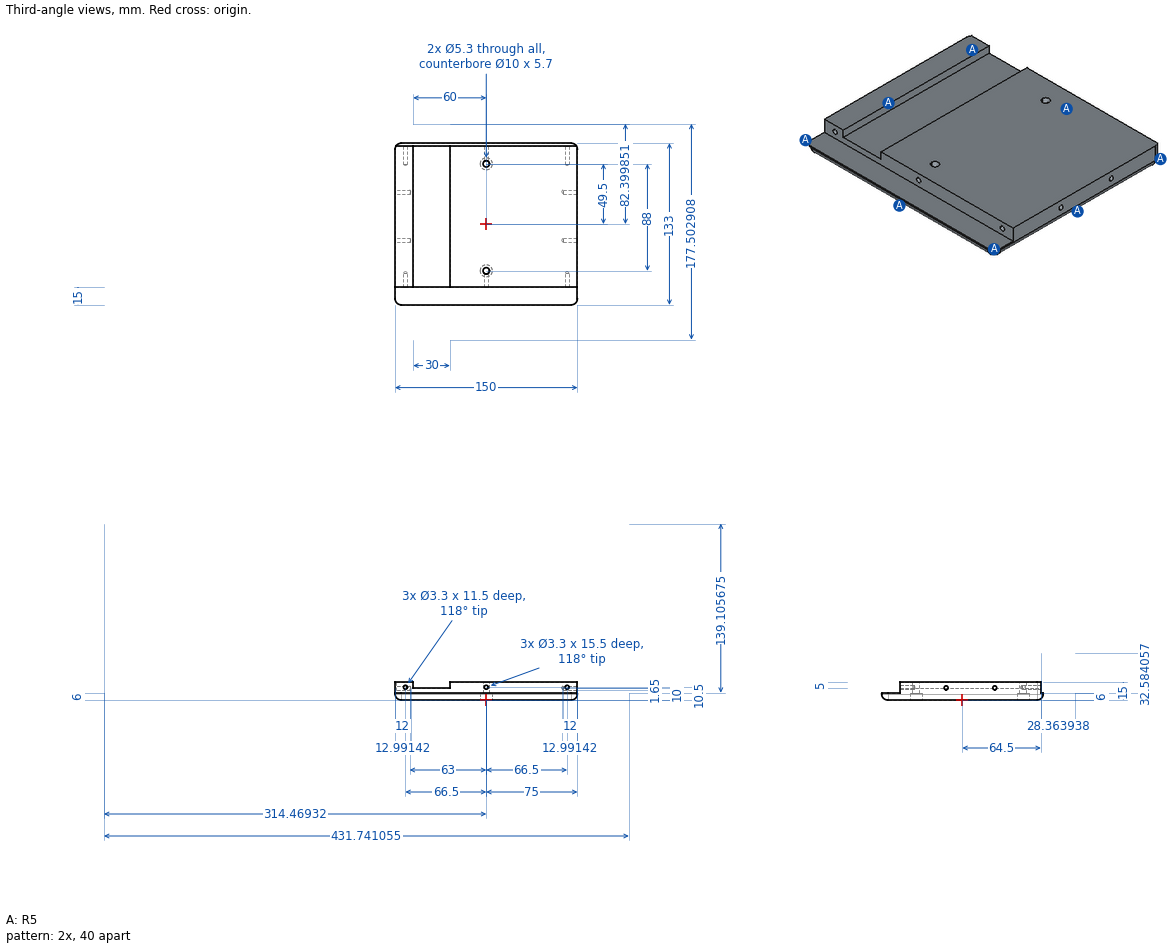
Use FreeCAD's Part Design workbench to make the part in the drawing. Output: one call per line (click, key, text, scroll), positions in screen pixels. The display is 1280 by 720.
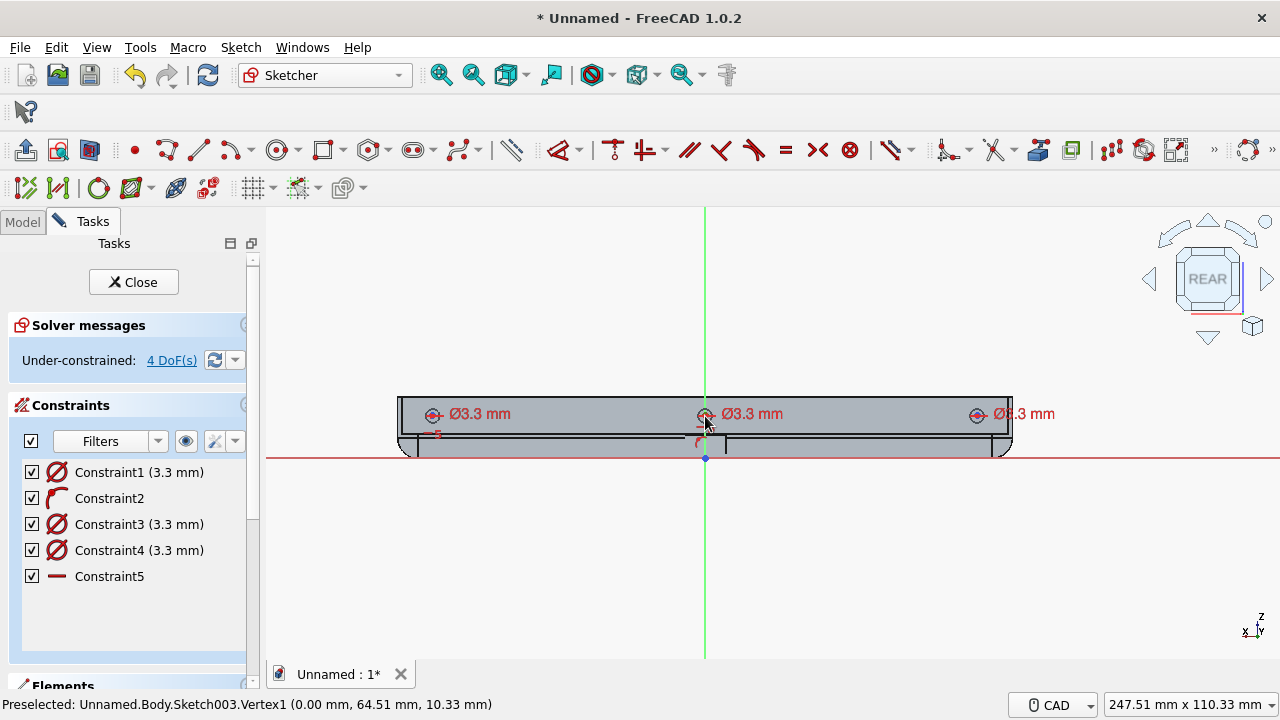
click(977, 416)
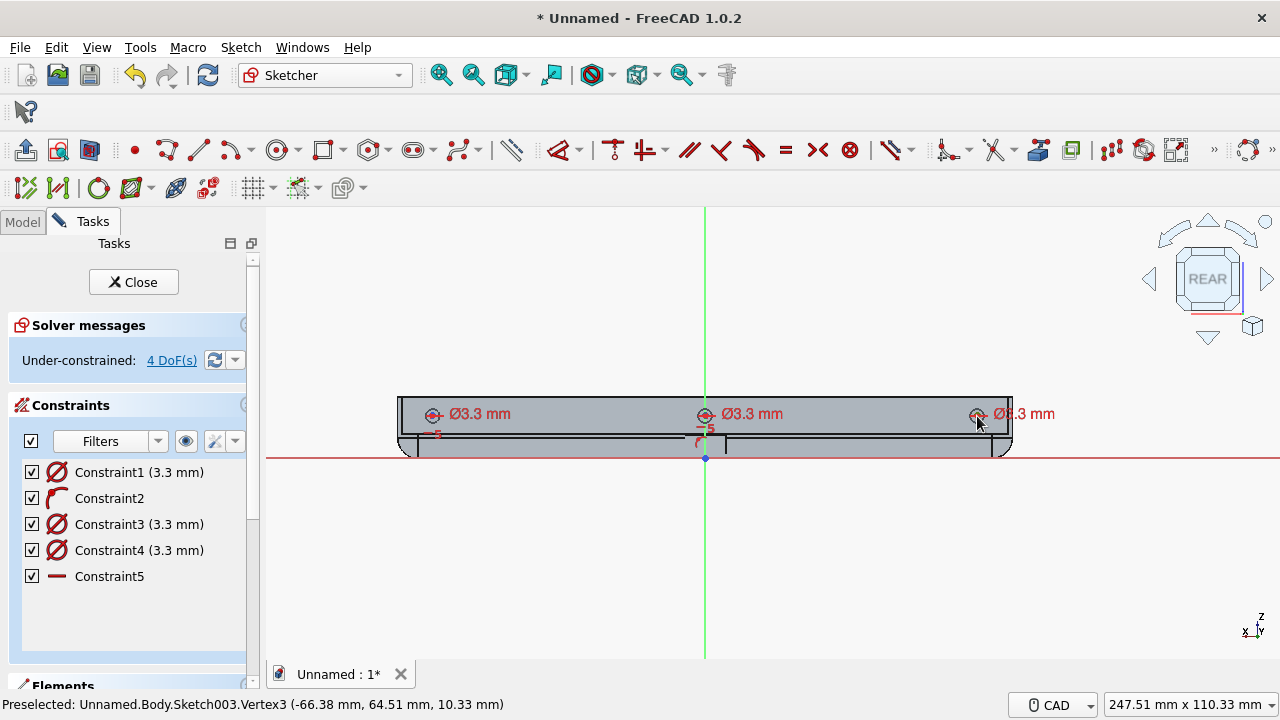
click(668, 150)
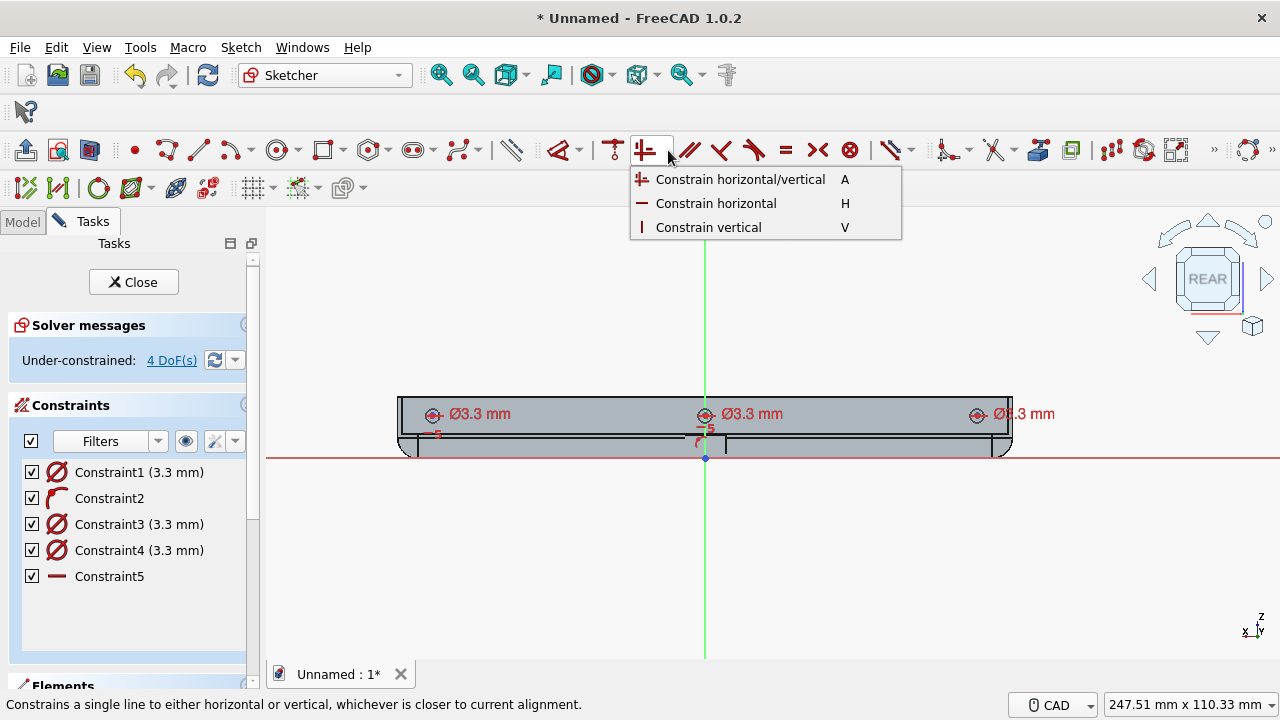
click(766, 203)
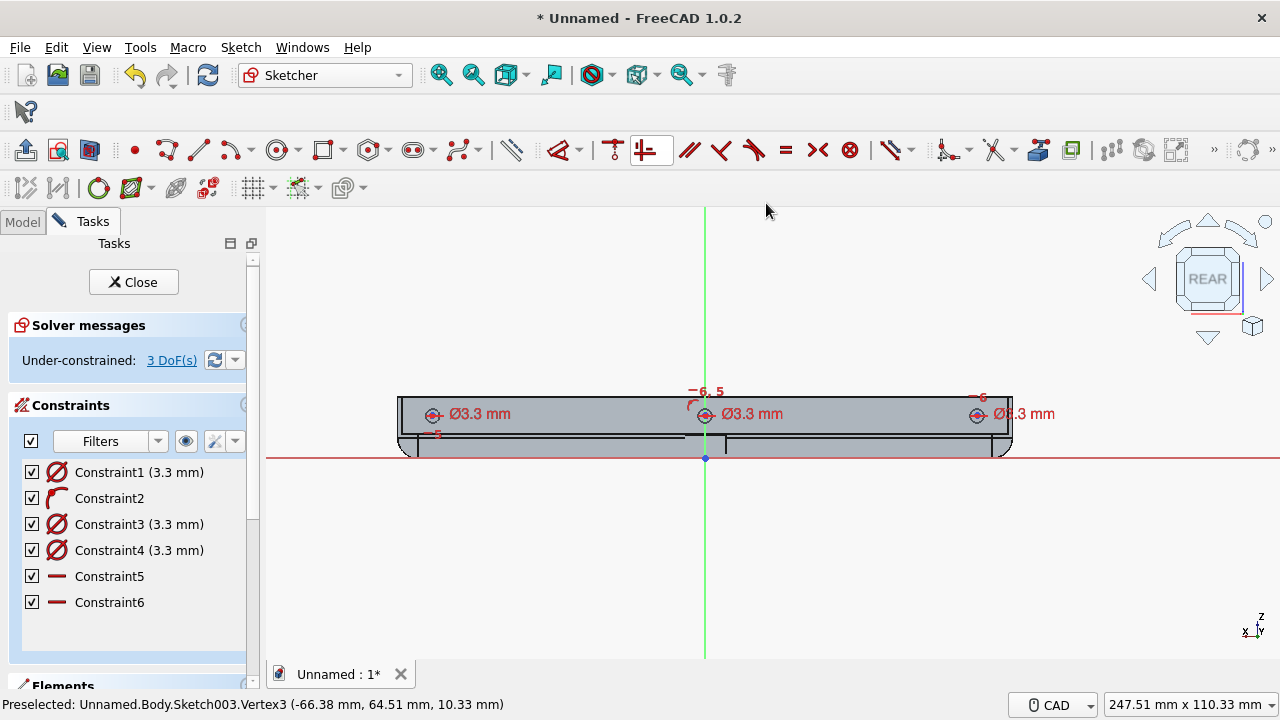
click(558, 150)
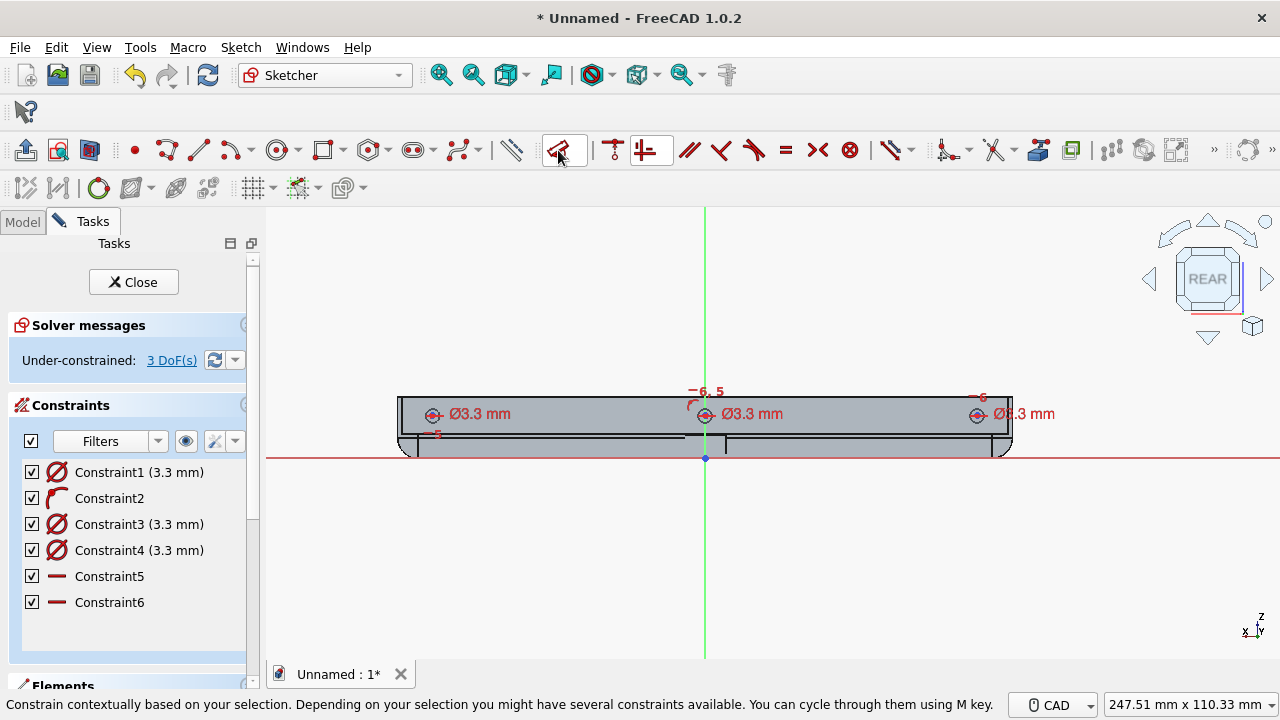
click(705, 416)
click(739, 437)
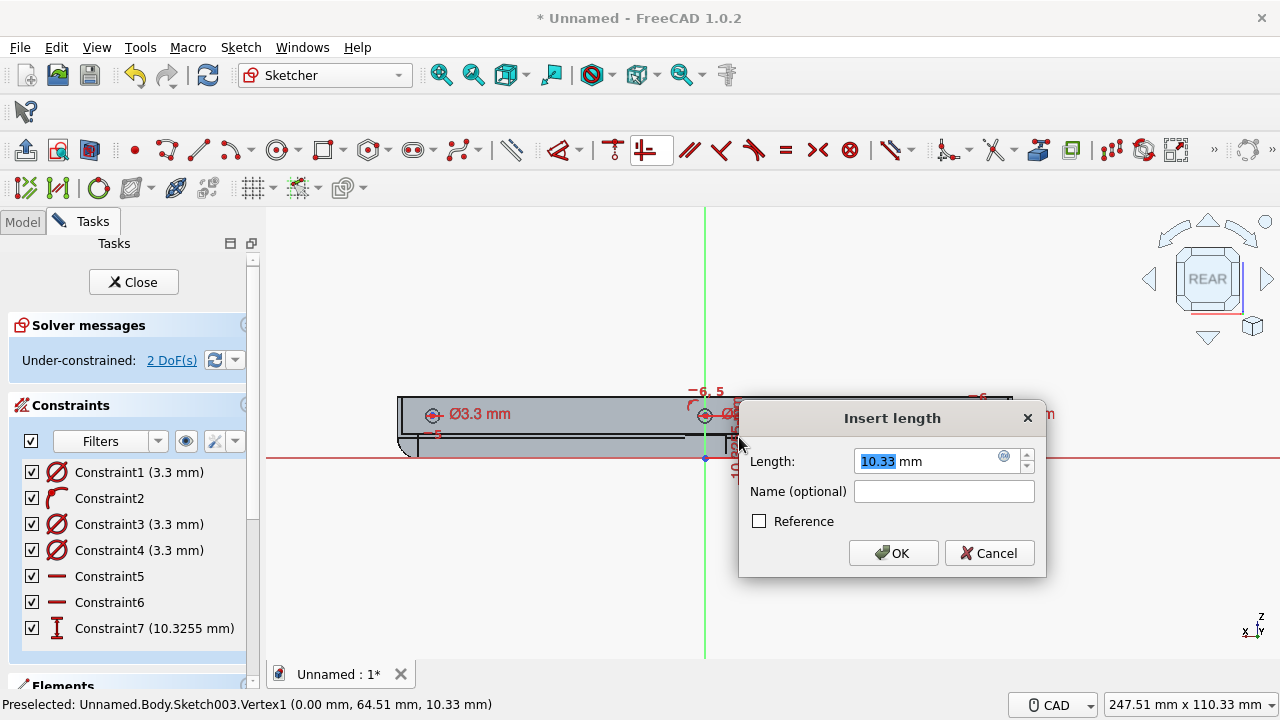
text(10.5)
key(Return)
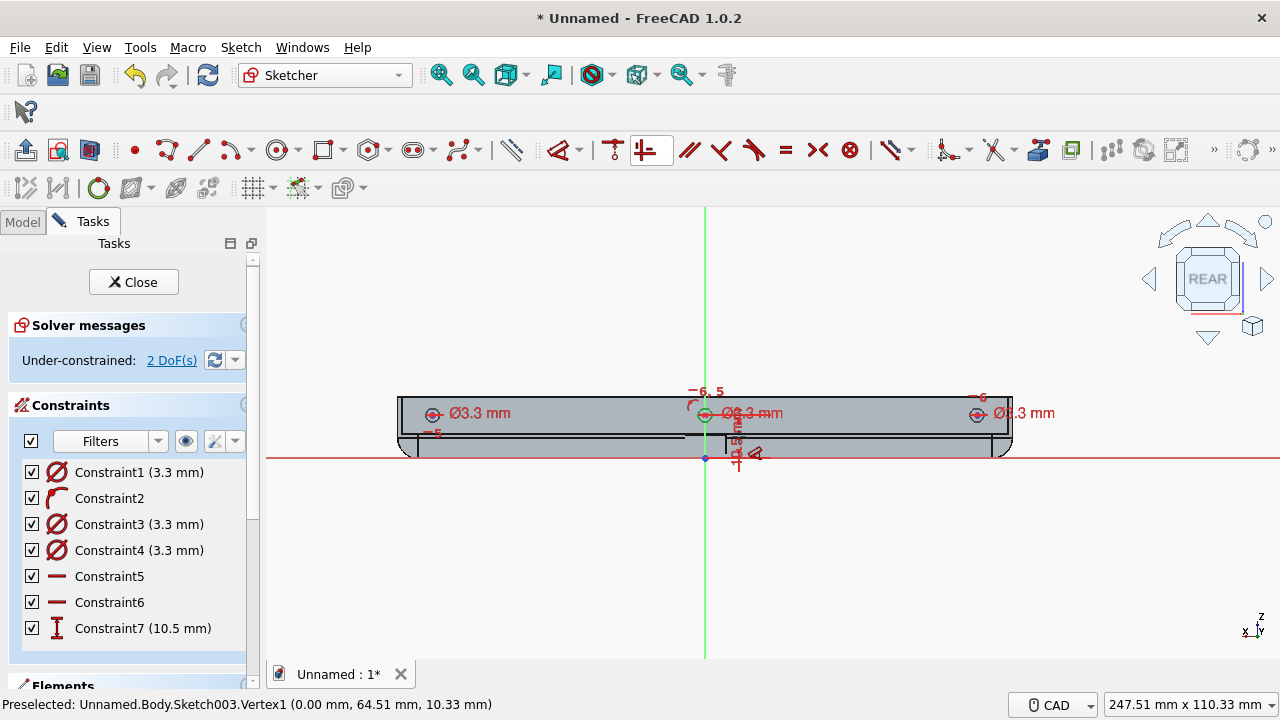
click(433, 415)
click(569, 492)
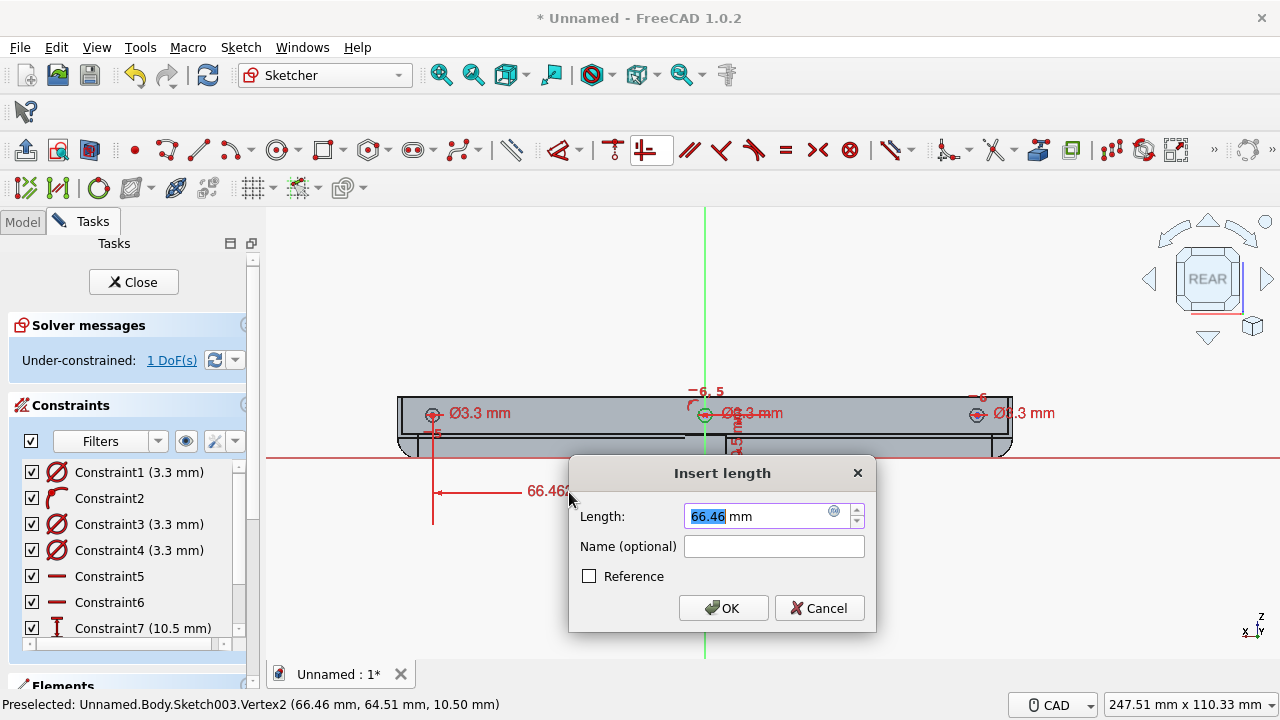
text(66.5)
key(Return)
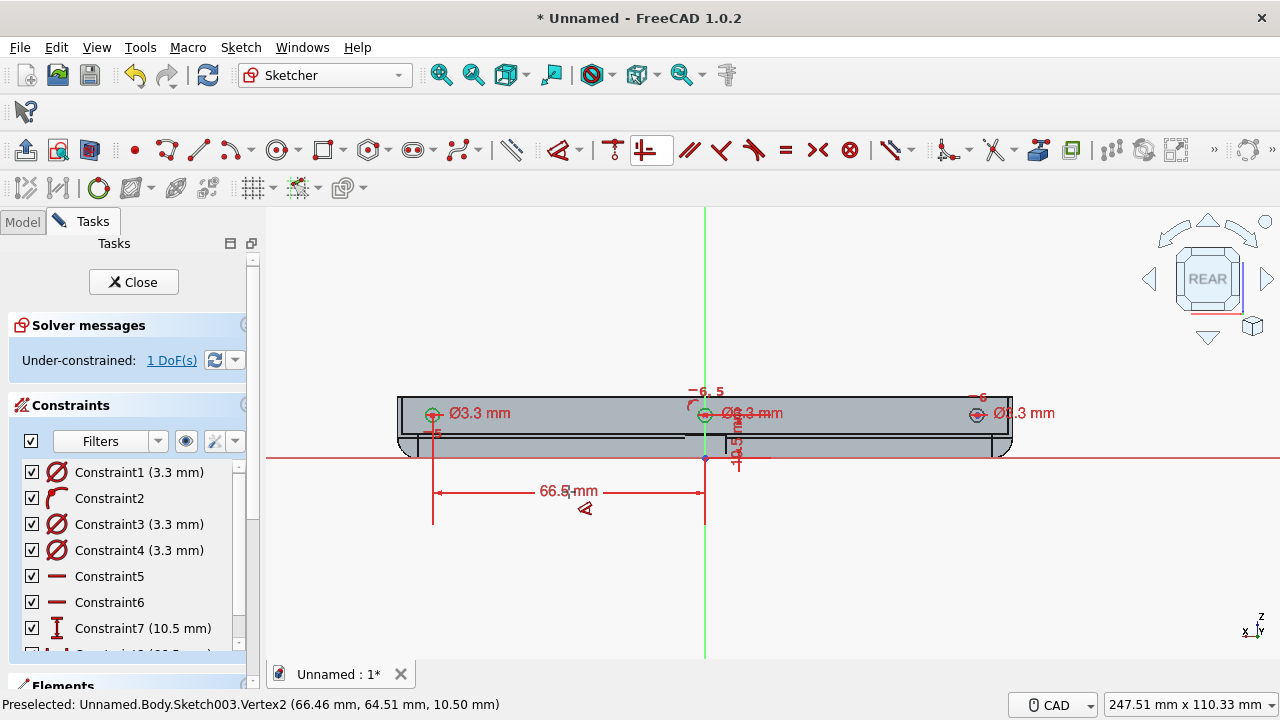
click(977, 415)
click(841, 492)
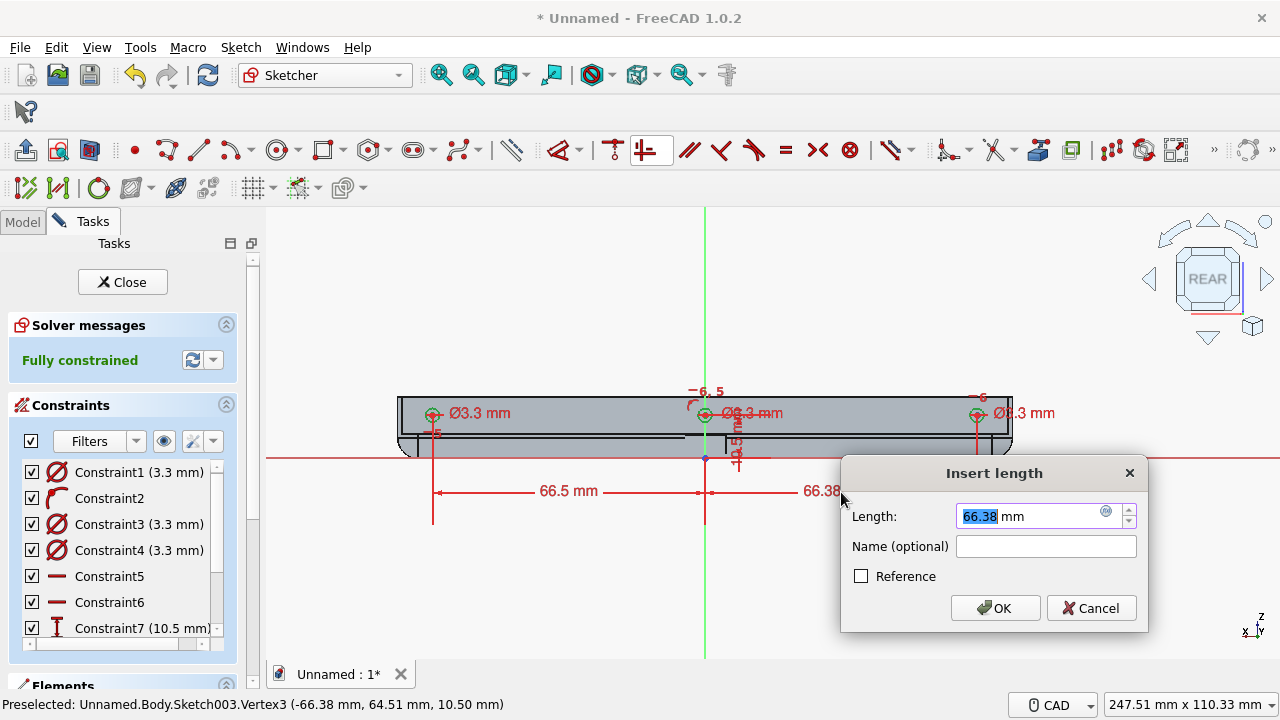
text(66.5)
key(Return)
key(Escape)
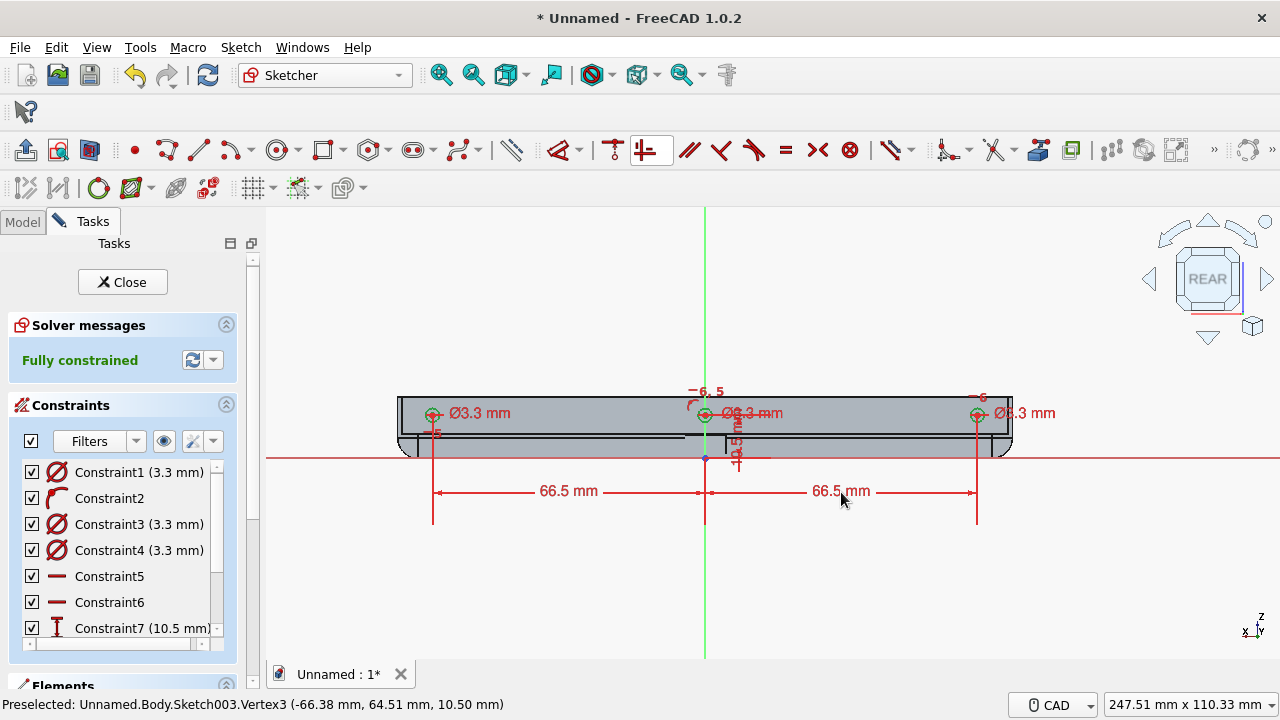
click(123, 282)